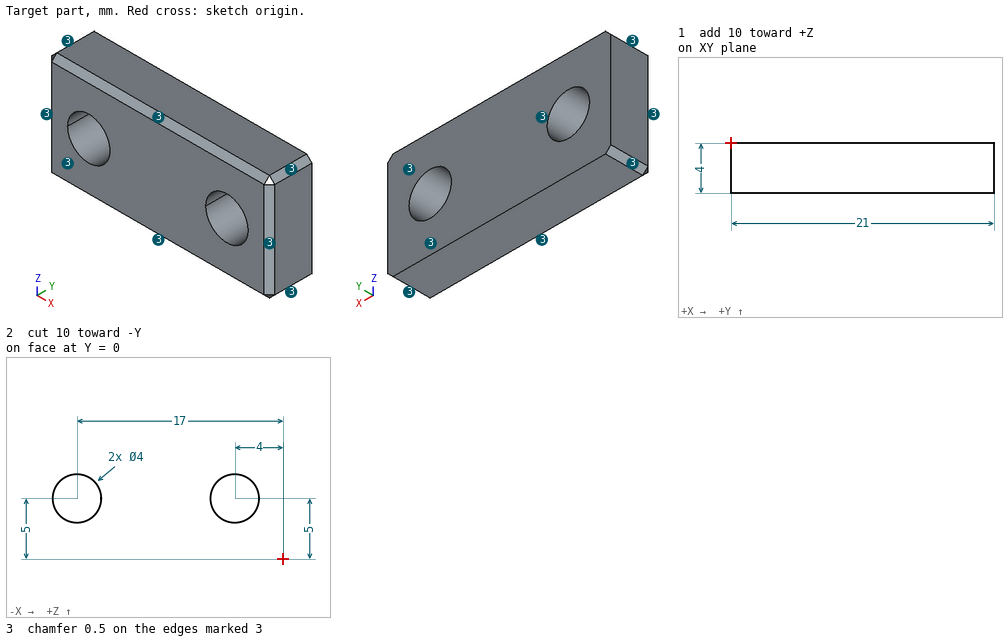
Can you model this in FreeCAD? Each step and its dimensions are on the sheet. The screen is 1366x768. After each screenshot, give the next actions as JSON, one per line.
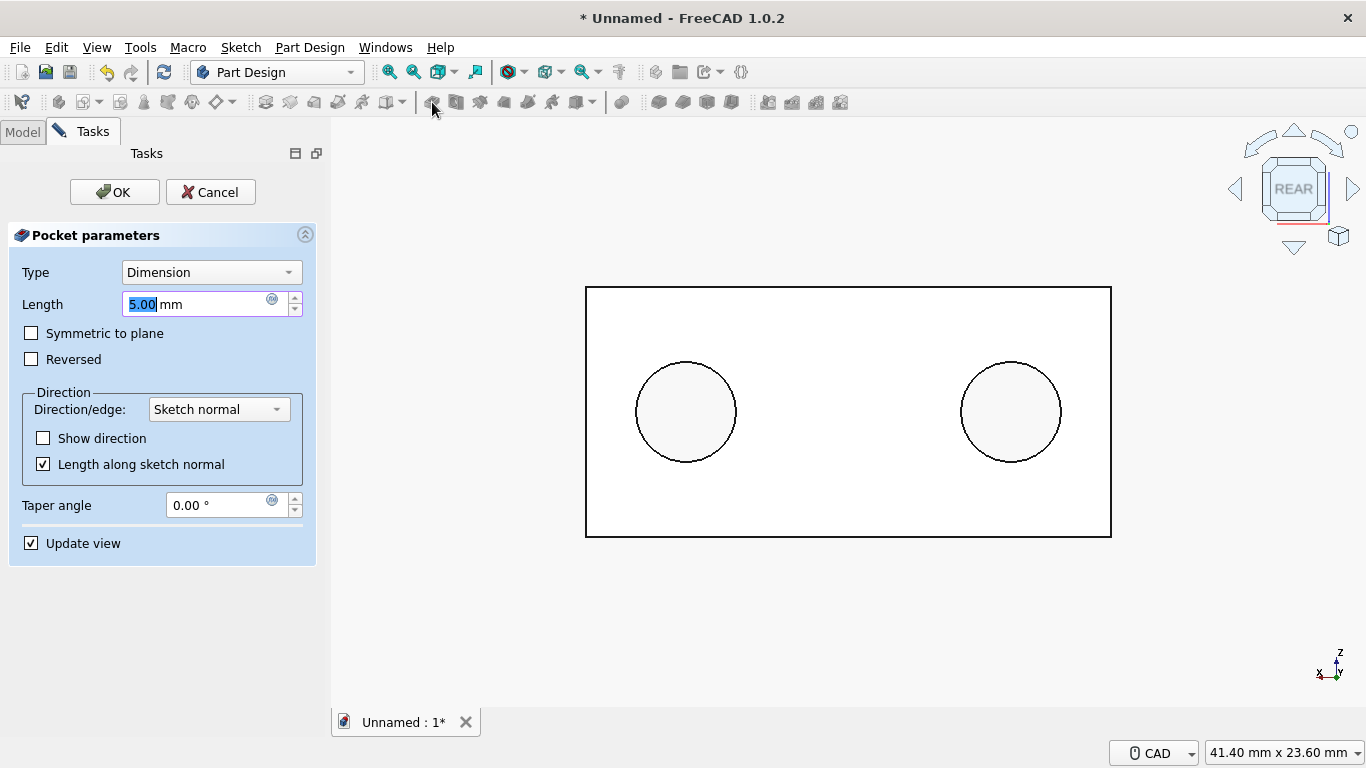
{"action": "type", "text": "10"}
{"action": "key", "text": "Tab"}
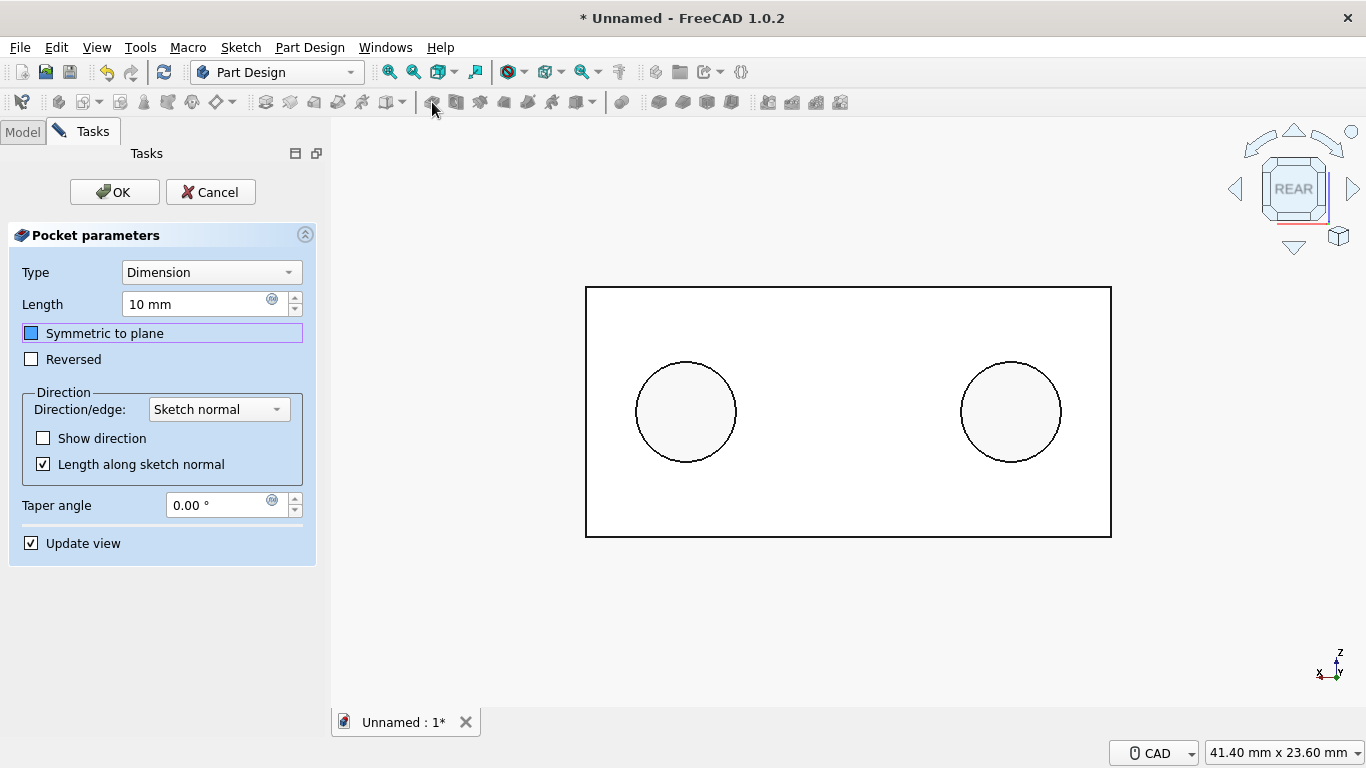
{"action": "left_click", "coordinate": [115, 192]}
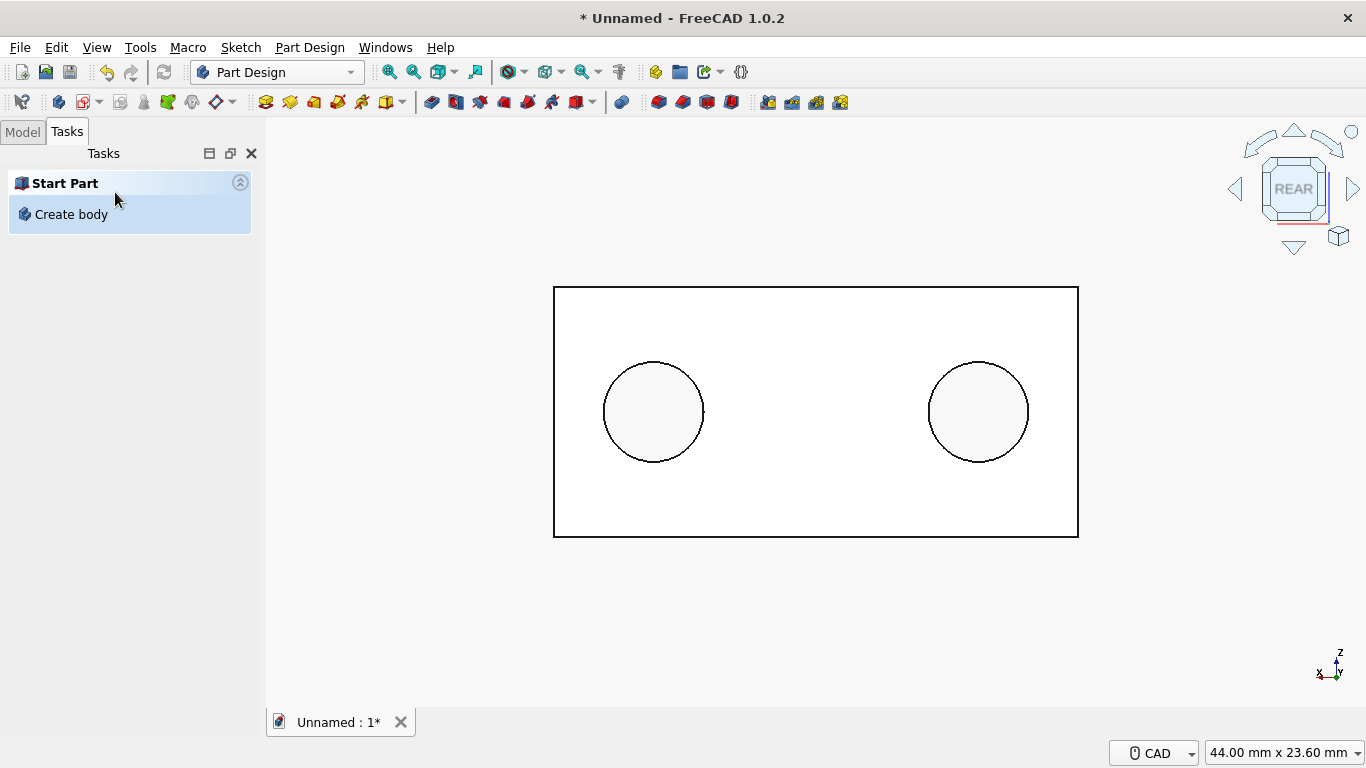
{"action": "key", "text": "0"}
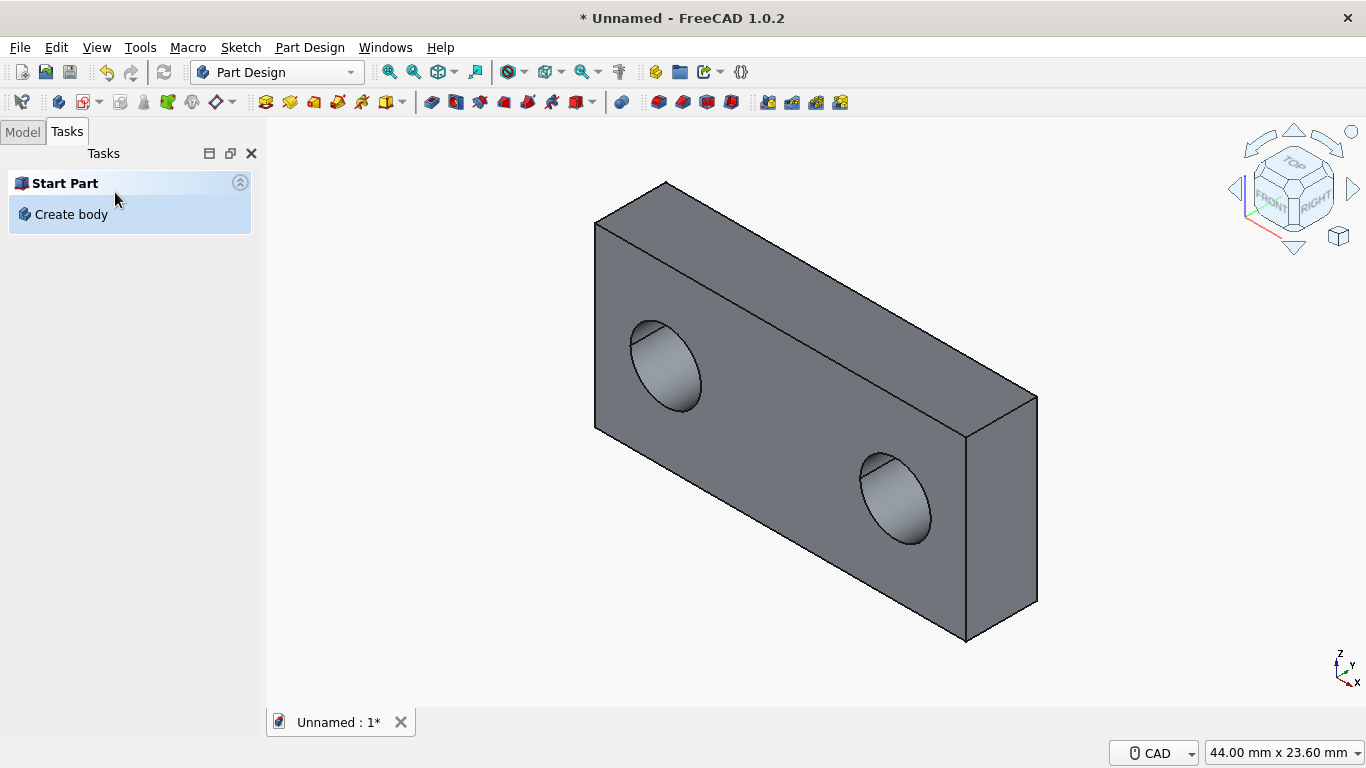
{"action": "left_click", "coordinate": [1002, 416]}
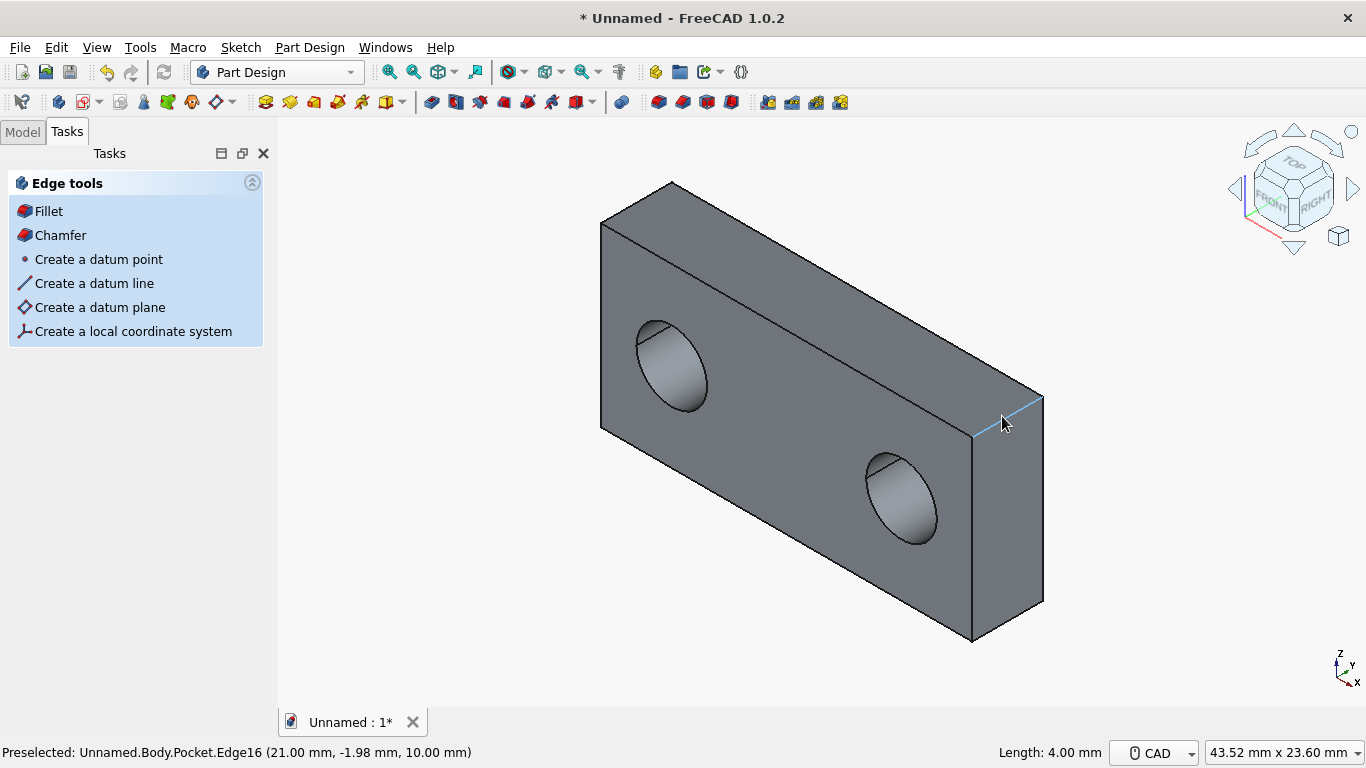
{"action": "left_click", "coordinate": [787, 329], "text": "ctrl"}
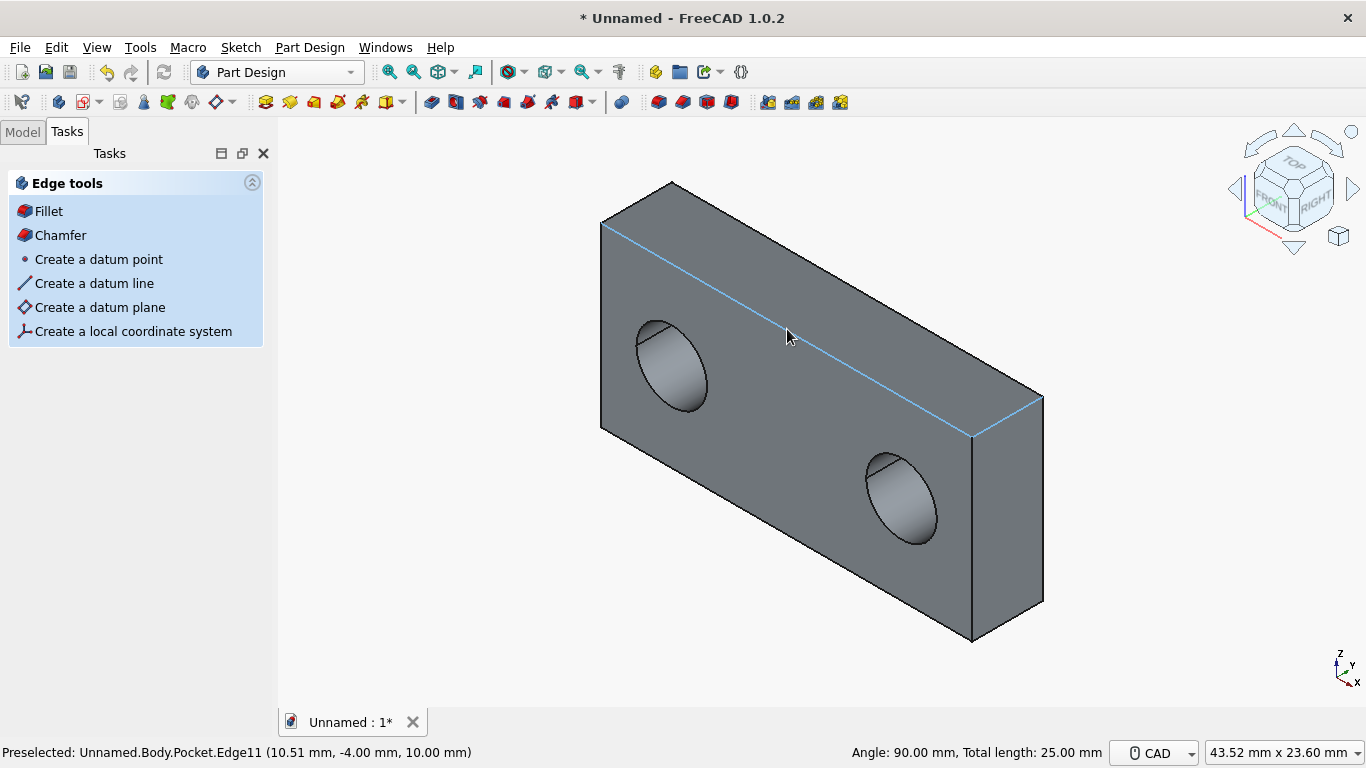
{"action": "left_click", "coordinate": [972, 539], "text": "ctrl"}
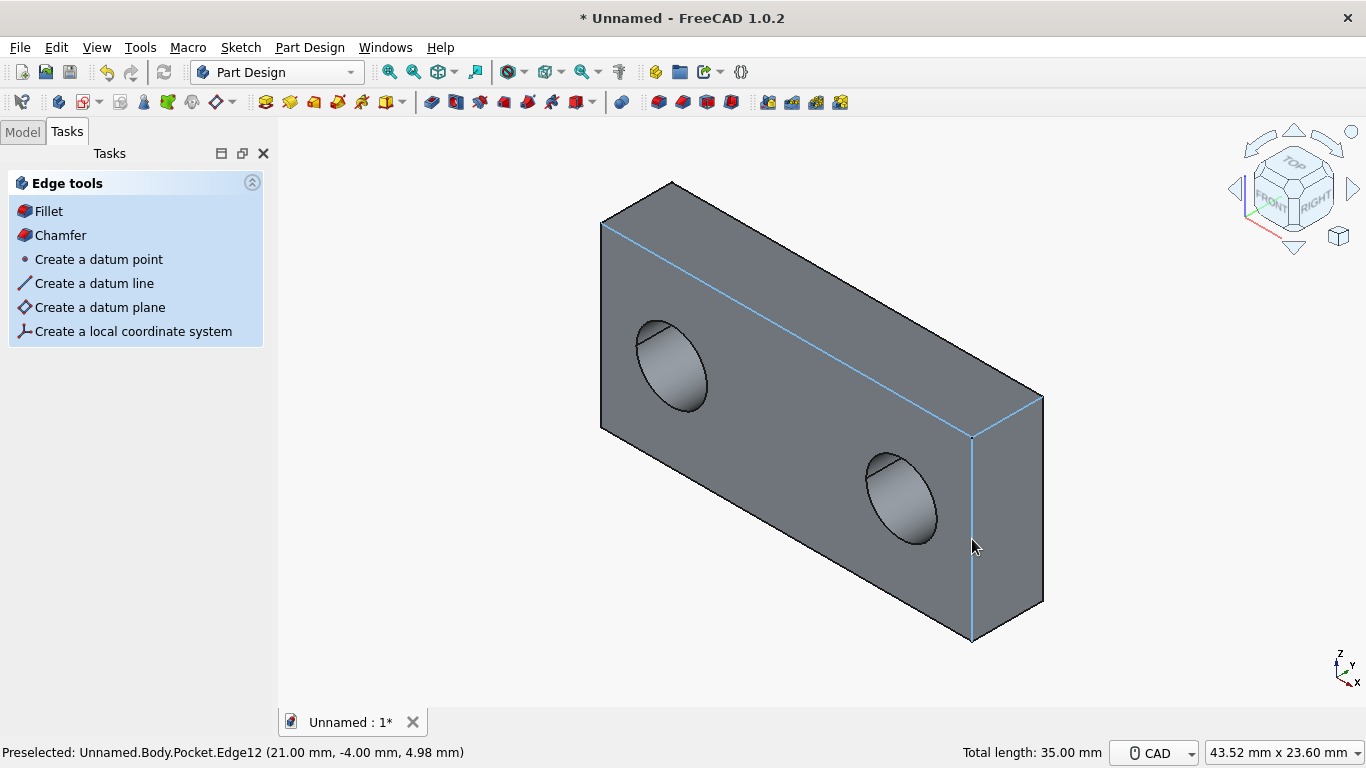
{"action": "key", "text": "2"}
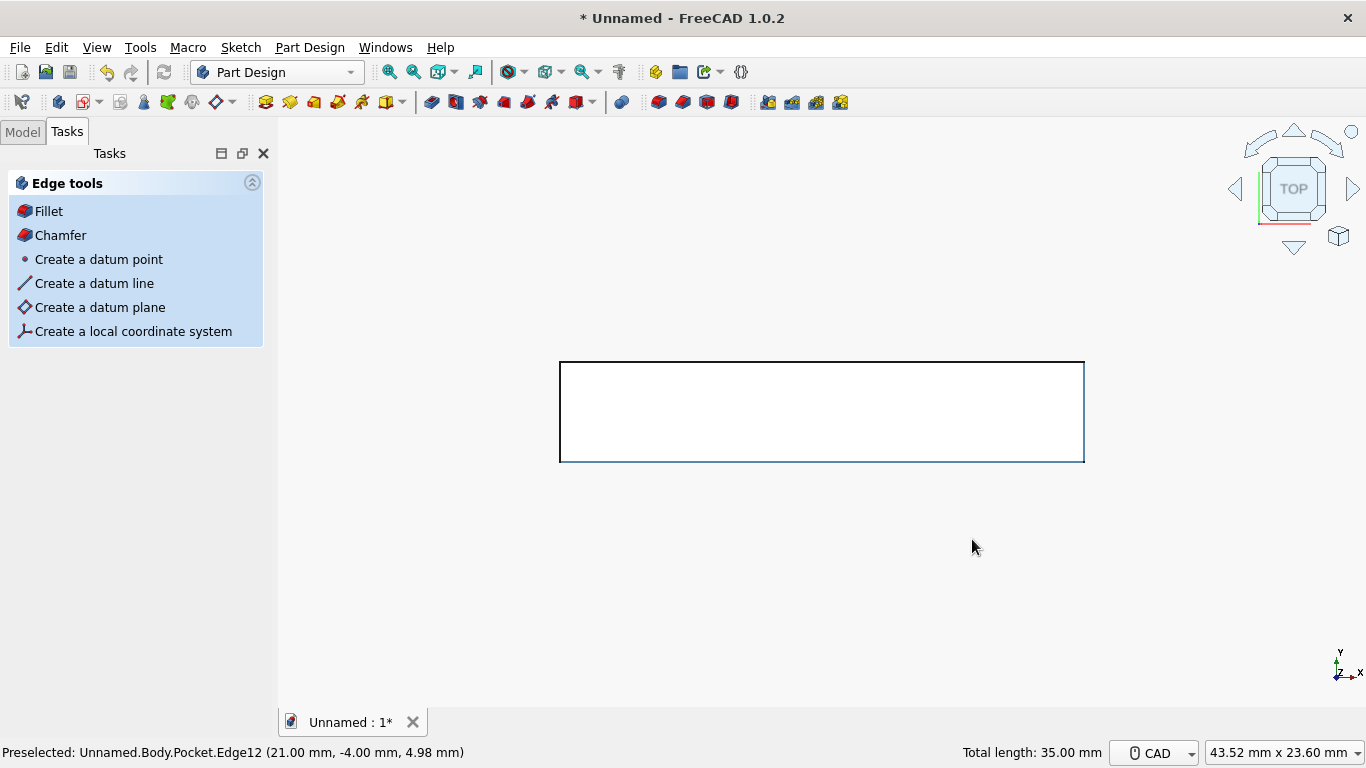
{"action": "left_click", "coordinate": [560, 411], "text": "ctrl"}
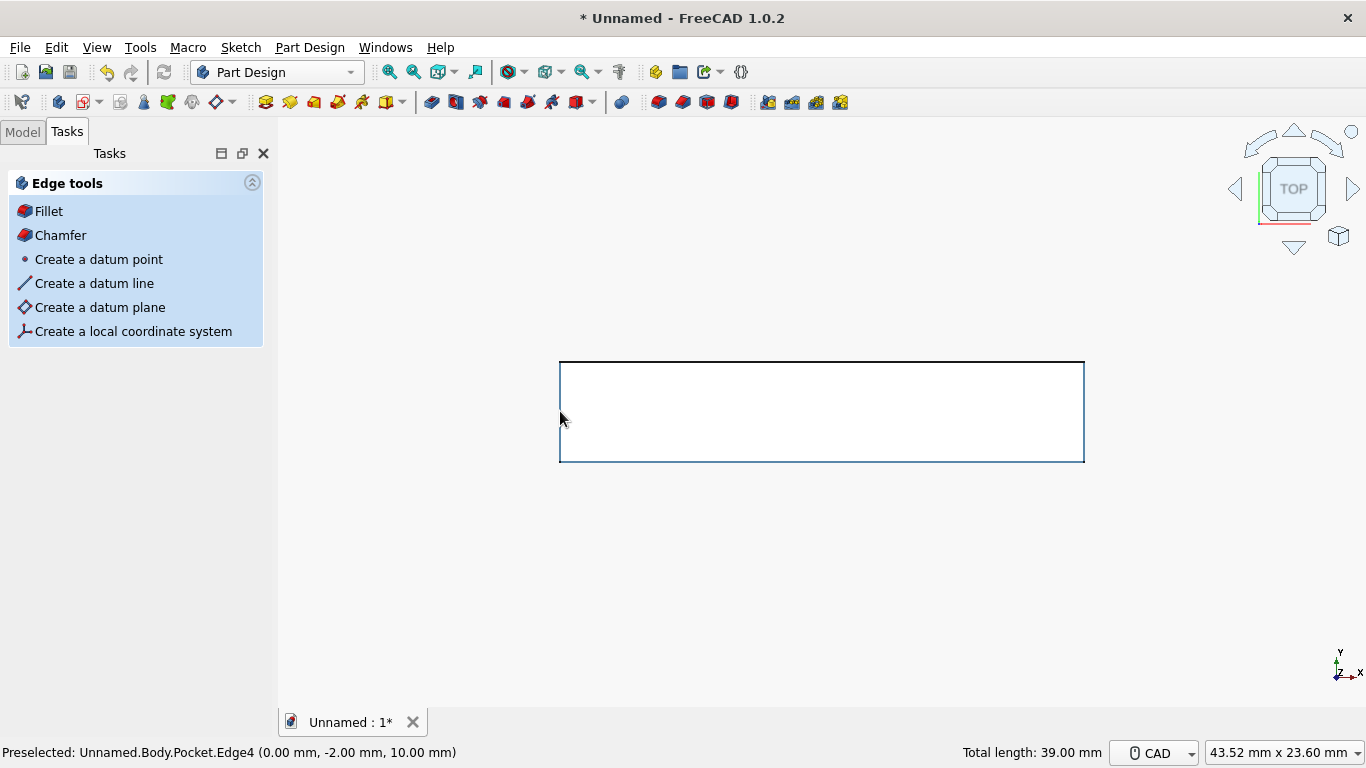
{"action": "key", "text": "1"}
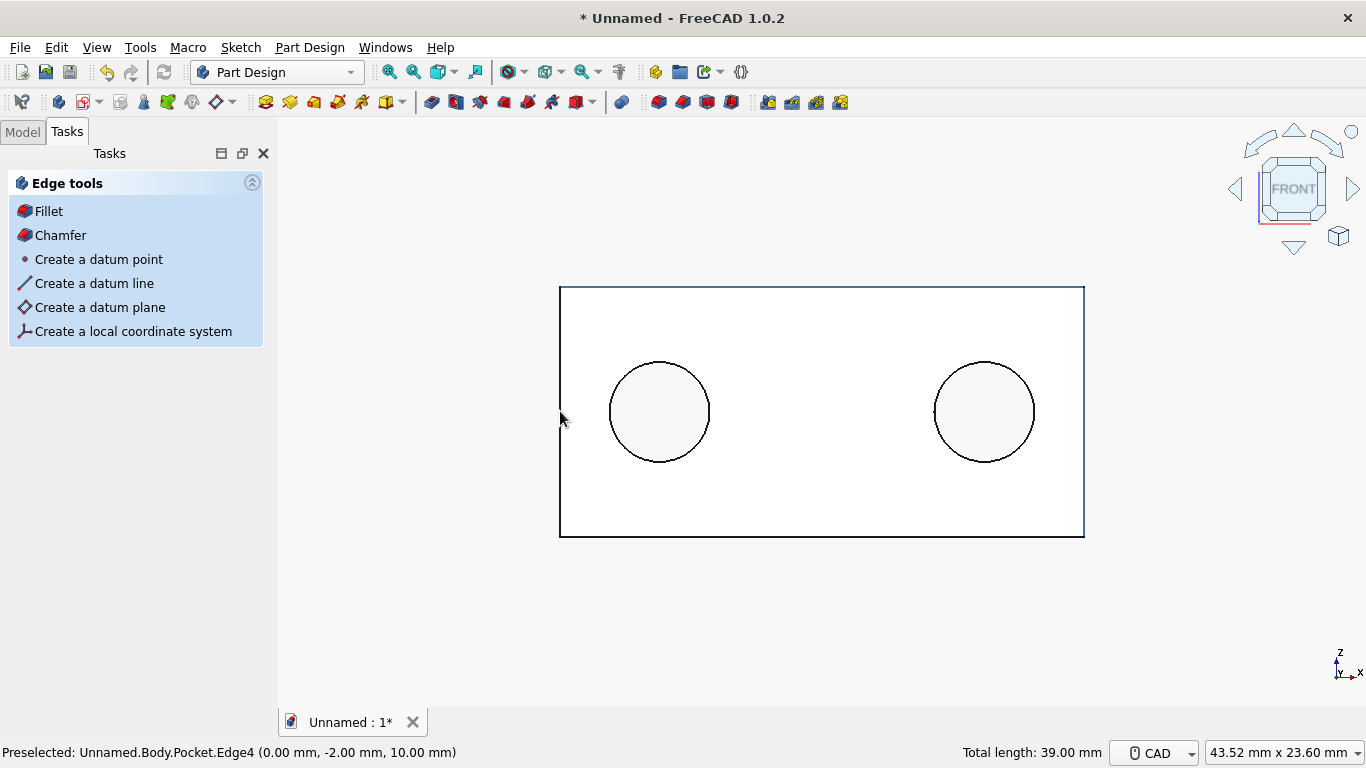
{"action": "left_click", "coordinate": [822, 536], "text": "ctrl"}